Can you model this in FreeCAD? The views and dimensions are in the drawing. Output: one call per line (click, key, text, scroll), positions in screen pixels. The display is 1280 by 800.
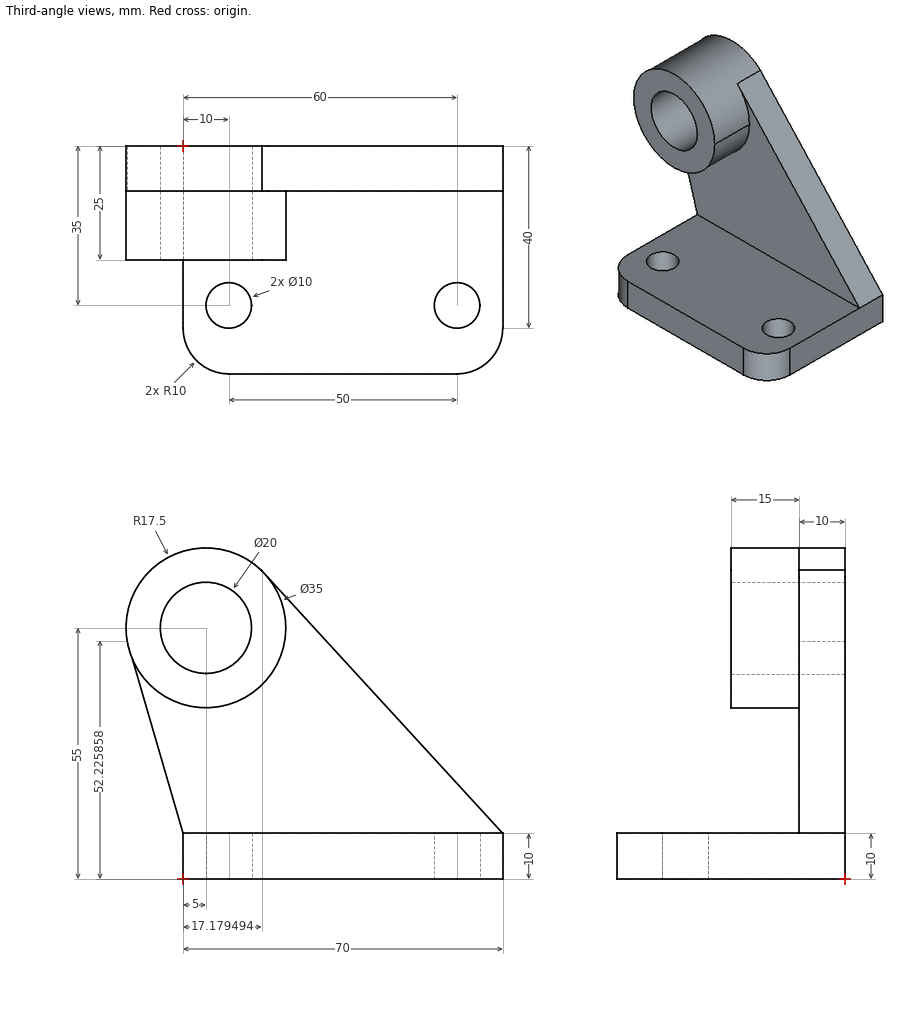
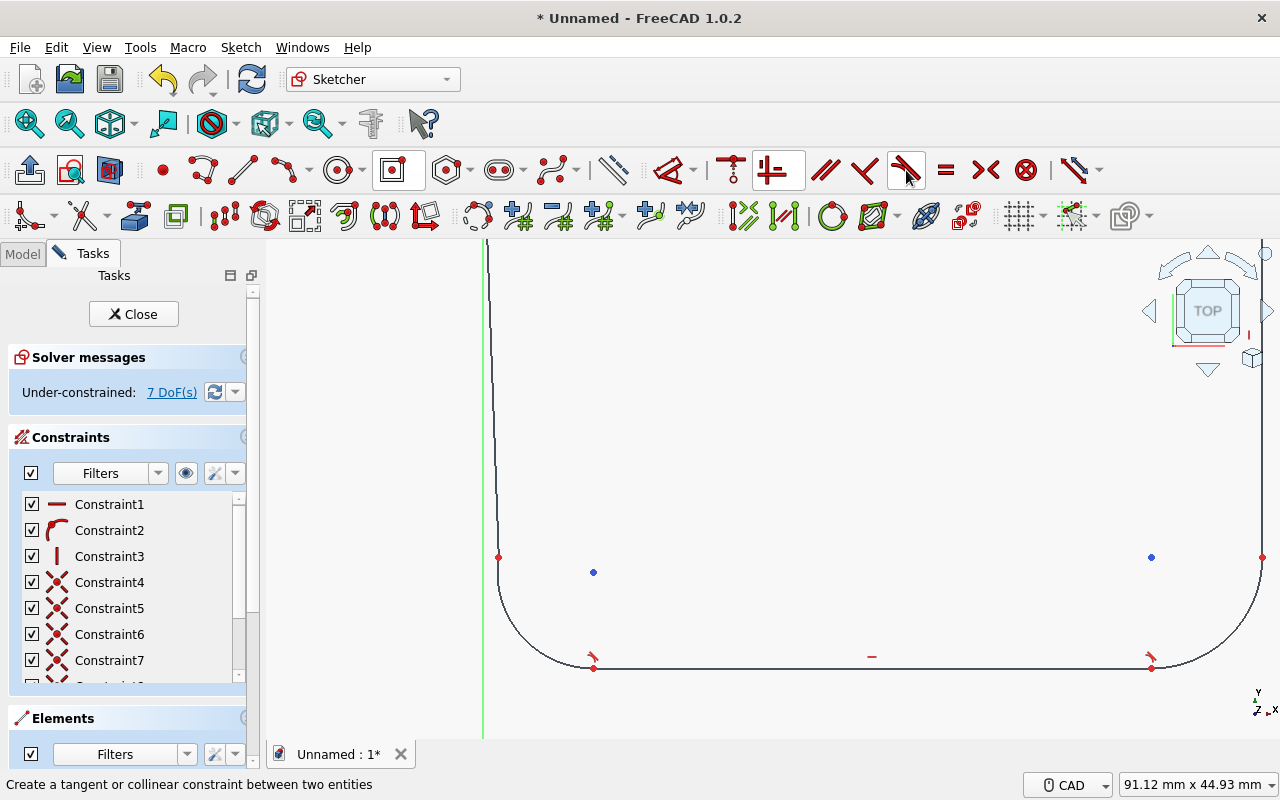
scroll(501, 610, down, 3)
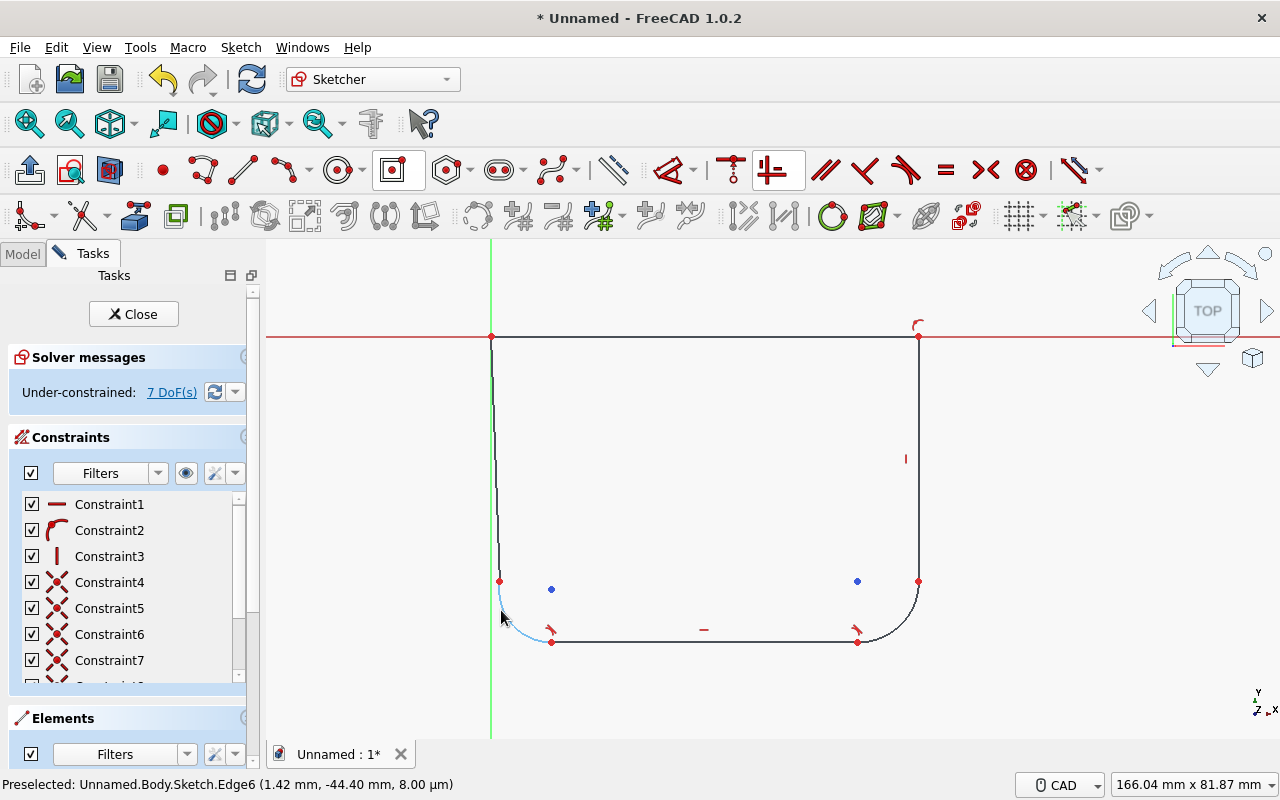
click(919, 508)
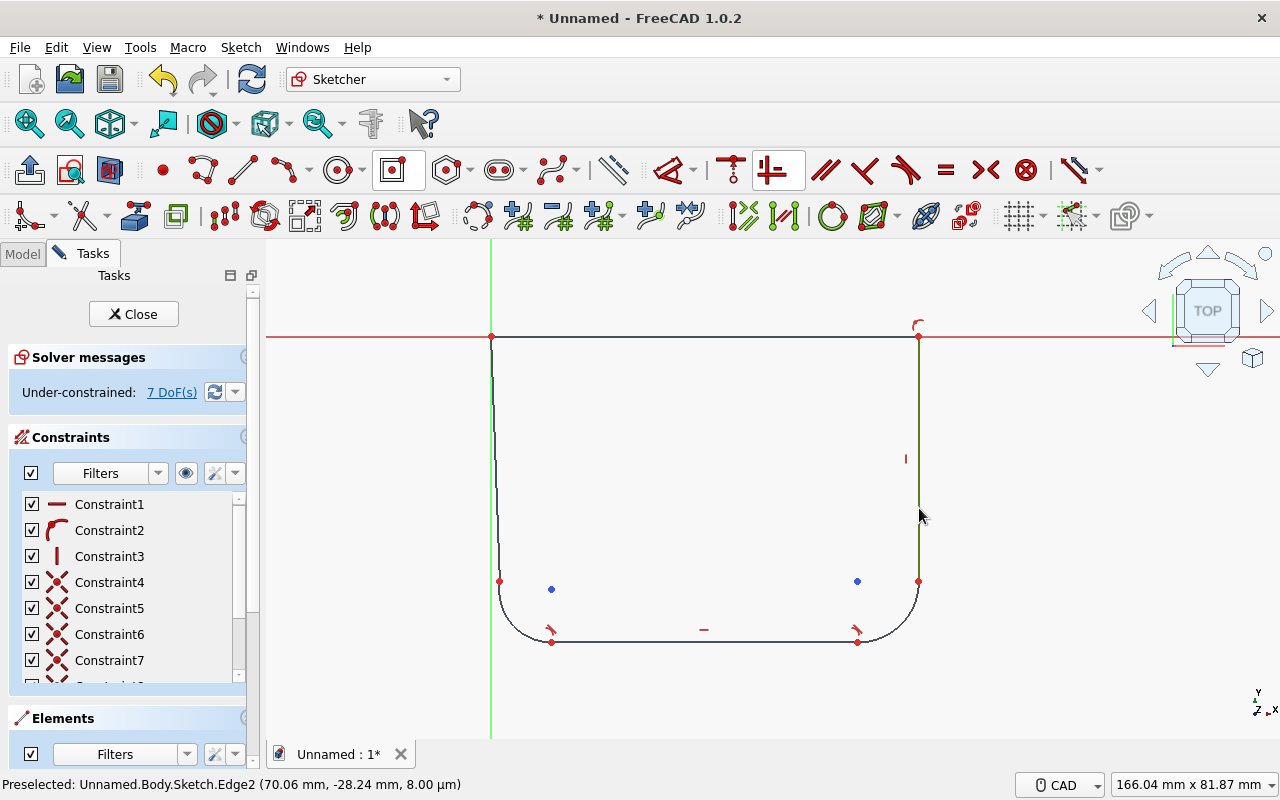
click(886, 636)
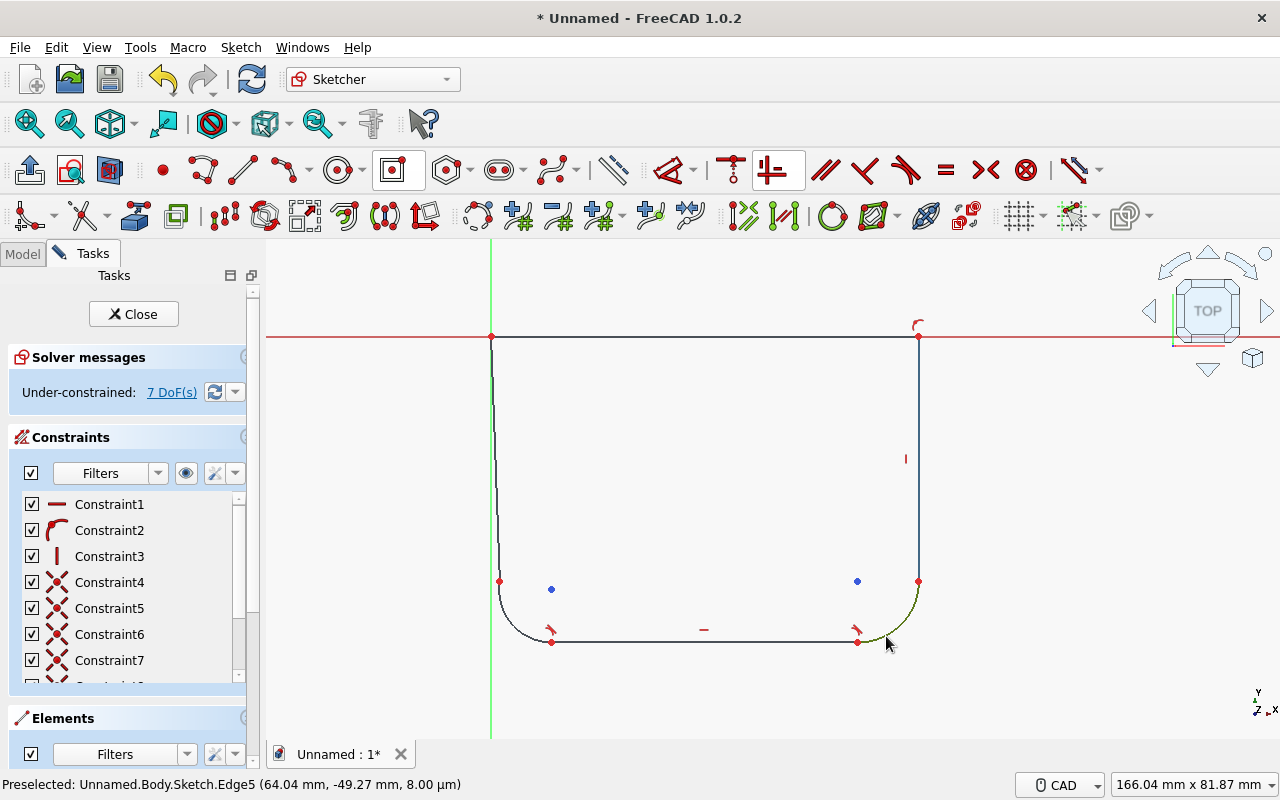
click(906, 170)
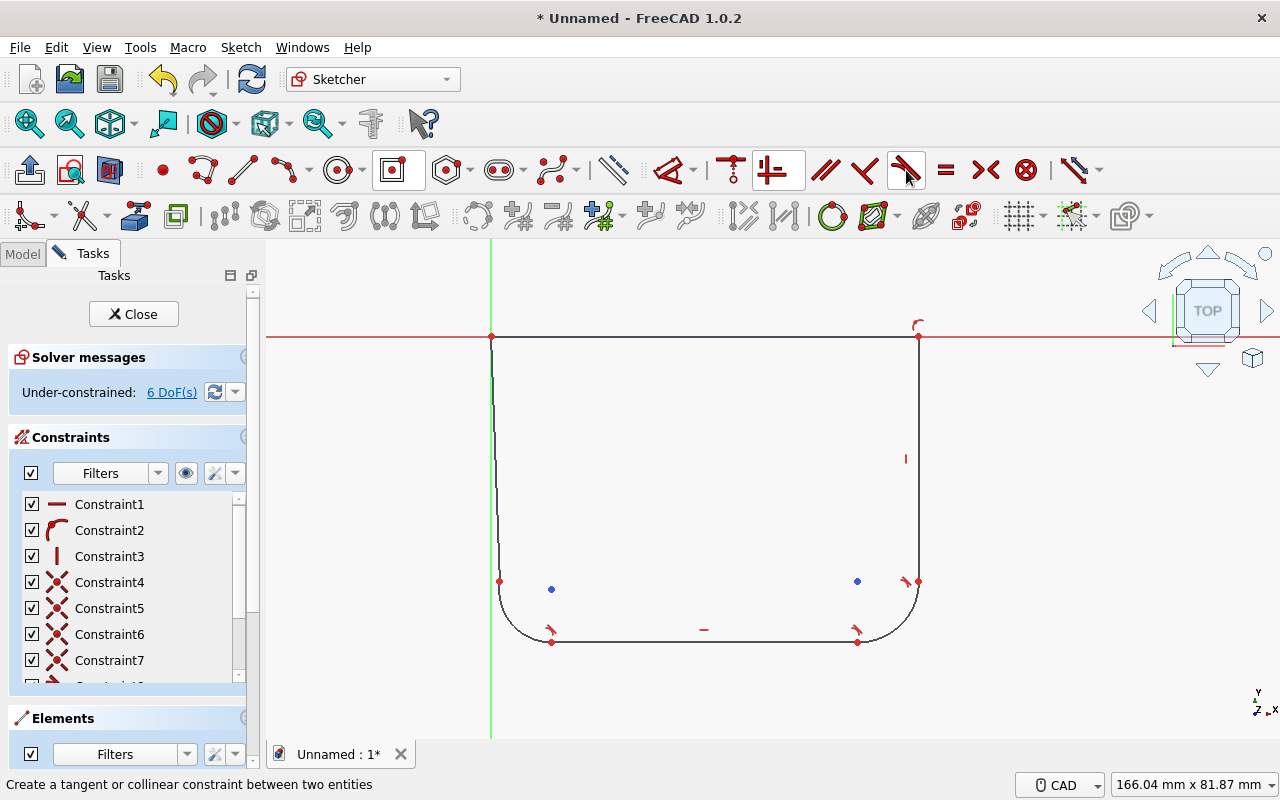
click(494, 410)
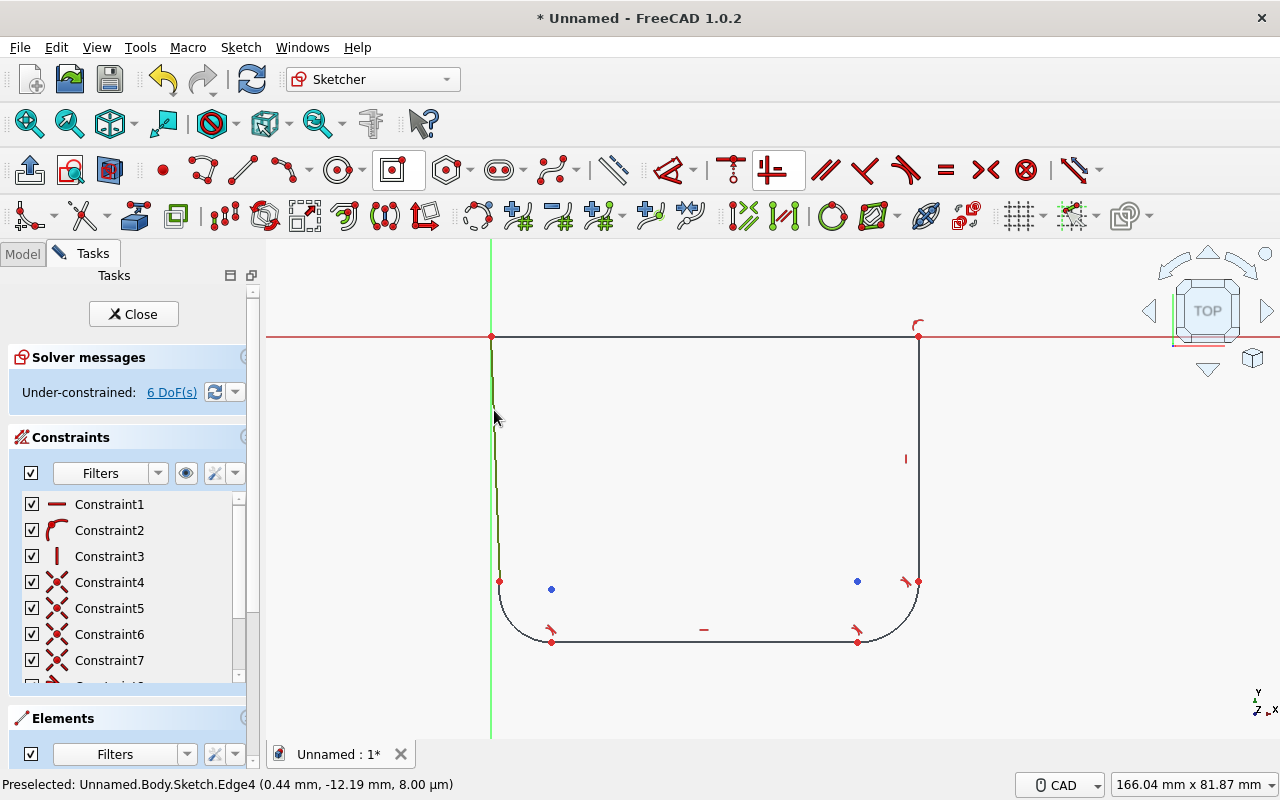
click(503, 608)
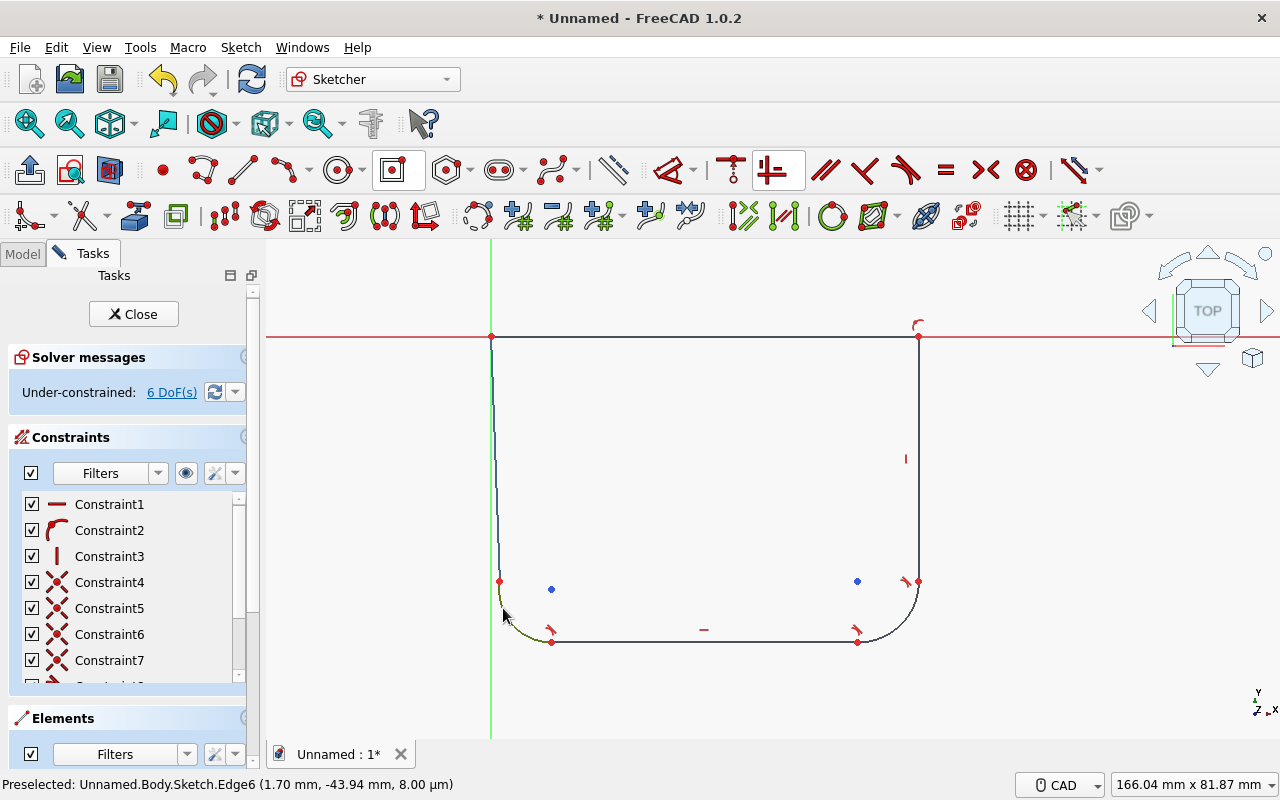
click(906, 170)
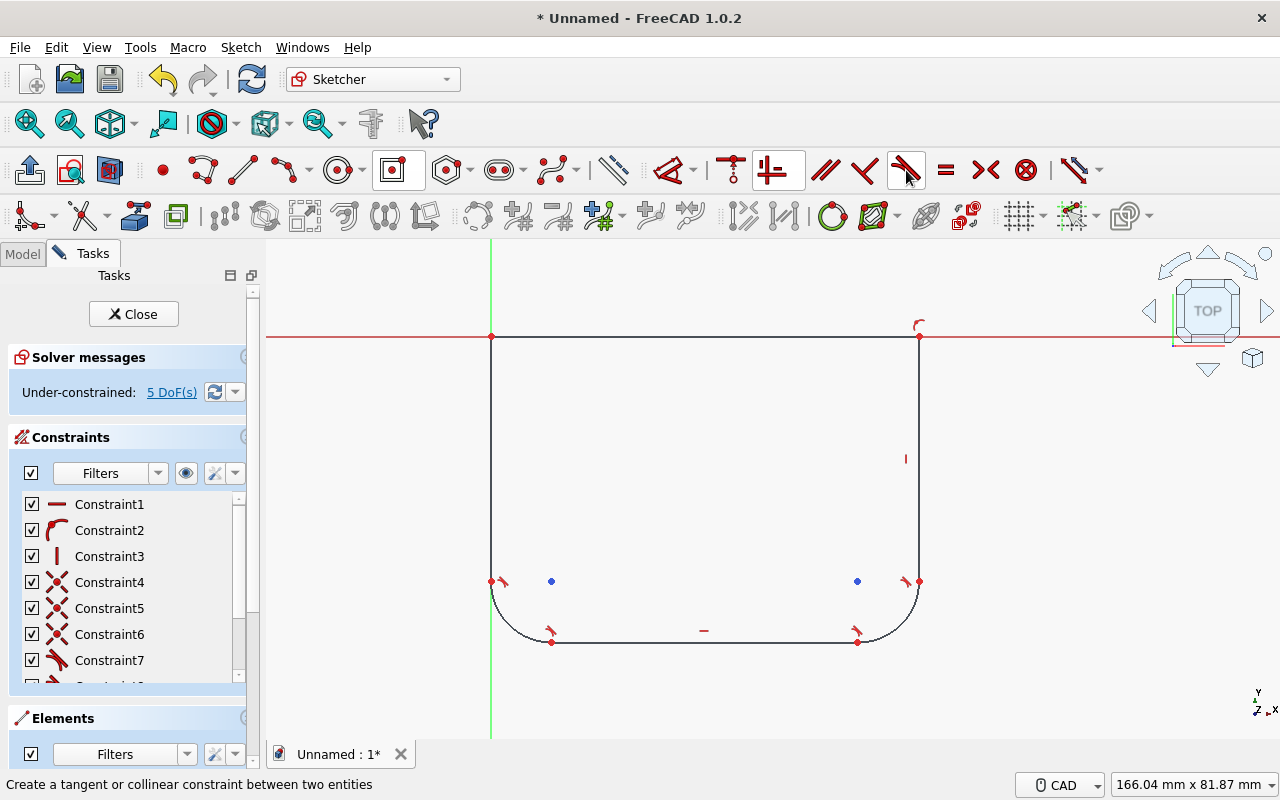
click(491, 410)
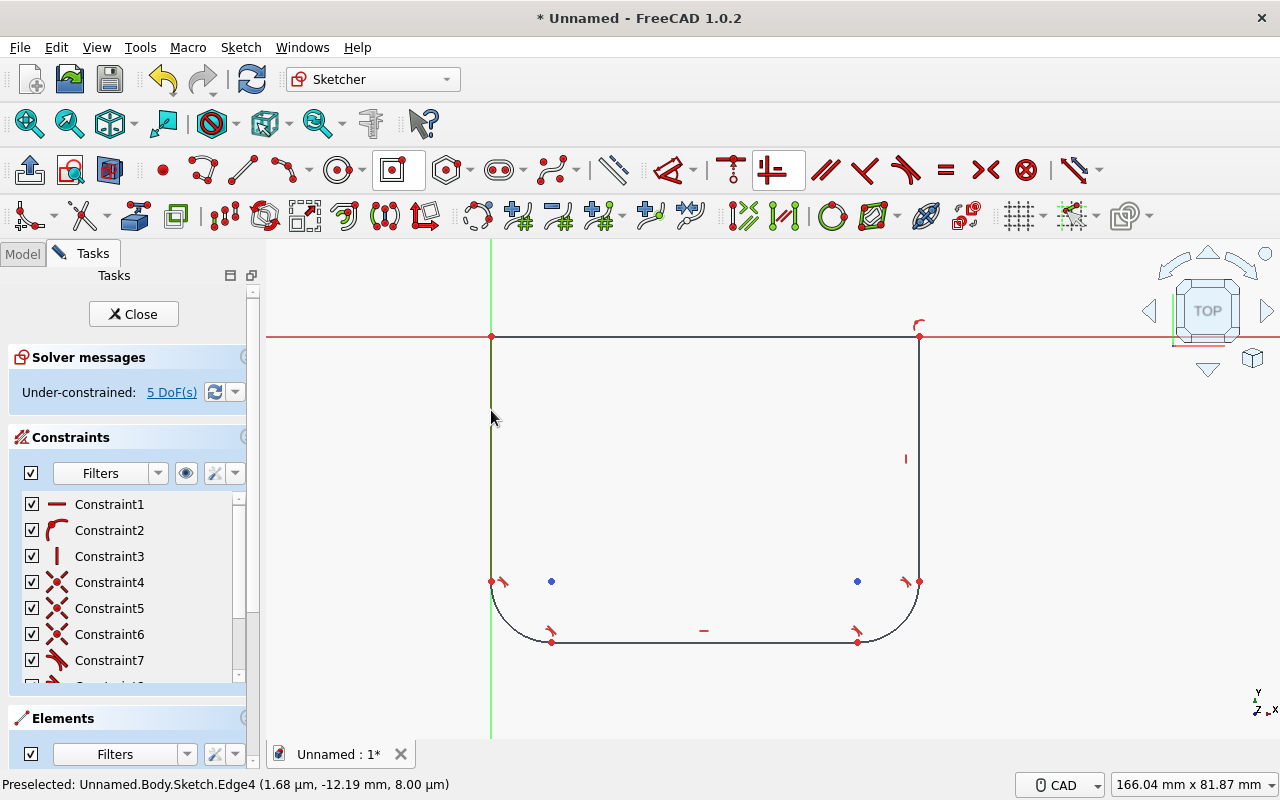
key(v)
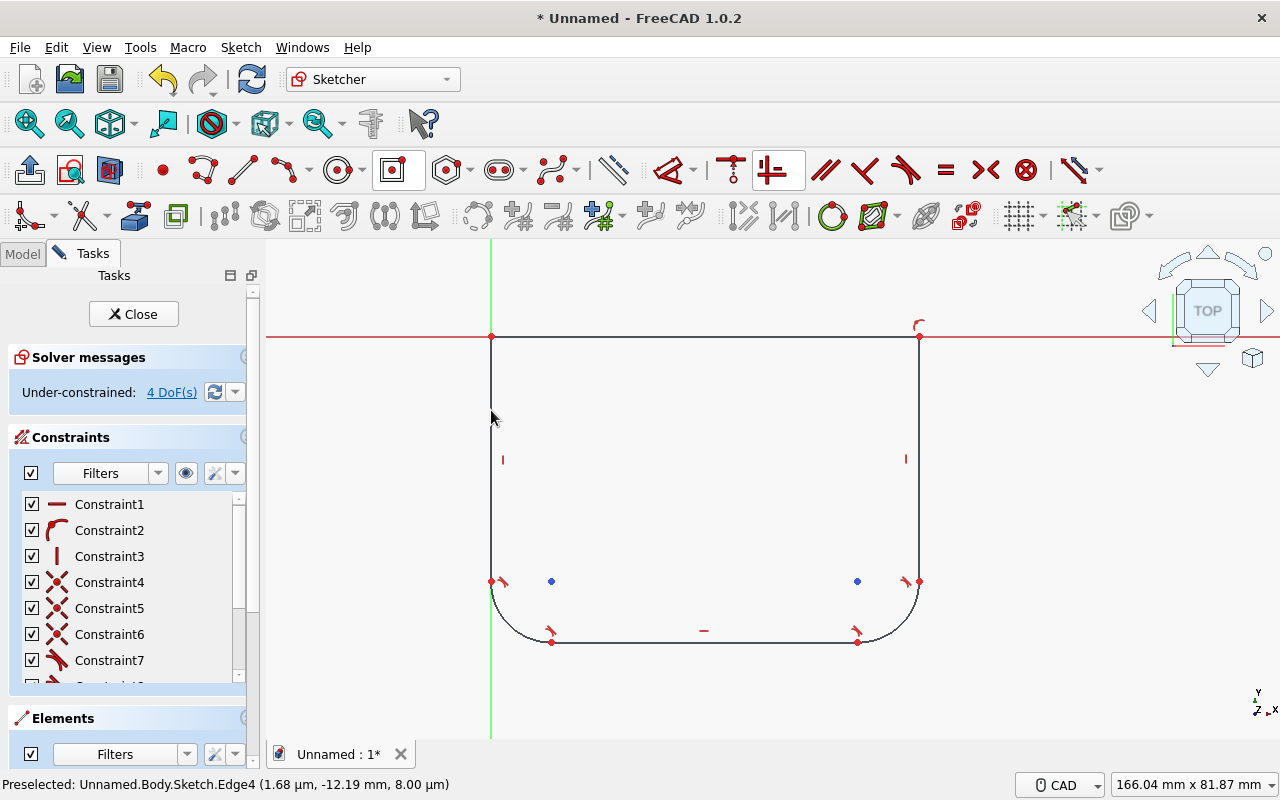
click(886, 636)